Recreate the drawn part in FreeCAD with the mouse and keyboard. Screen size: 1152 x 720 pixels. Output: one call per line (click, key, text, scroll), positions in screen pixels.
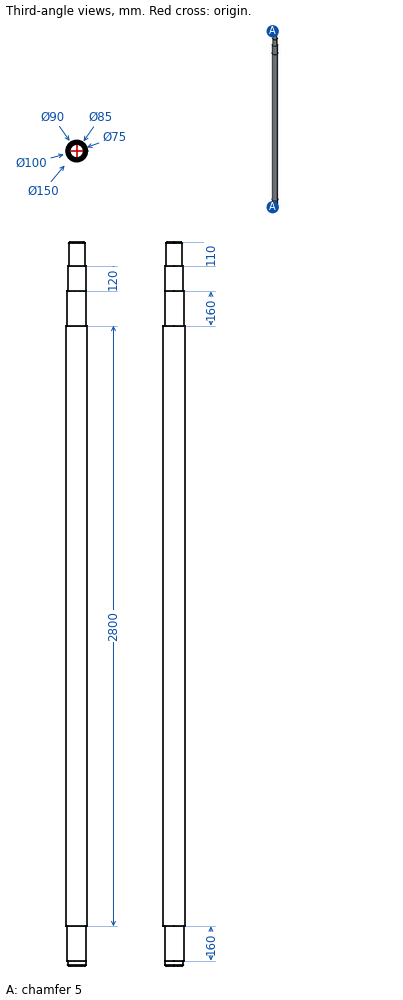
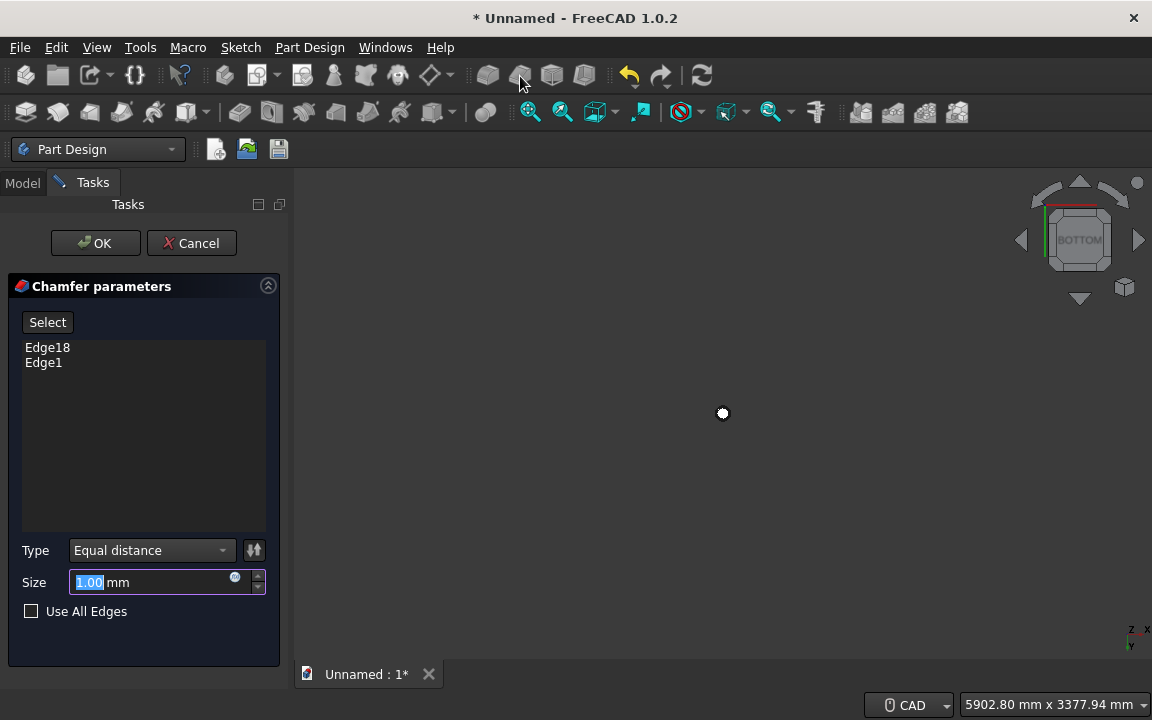
text(5)
key(Tab)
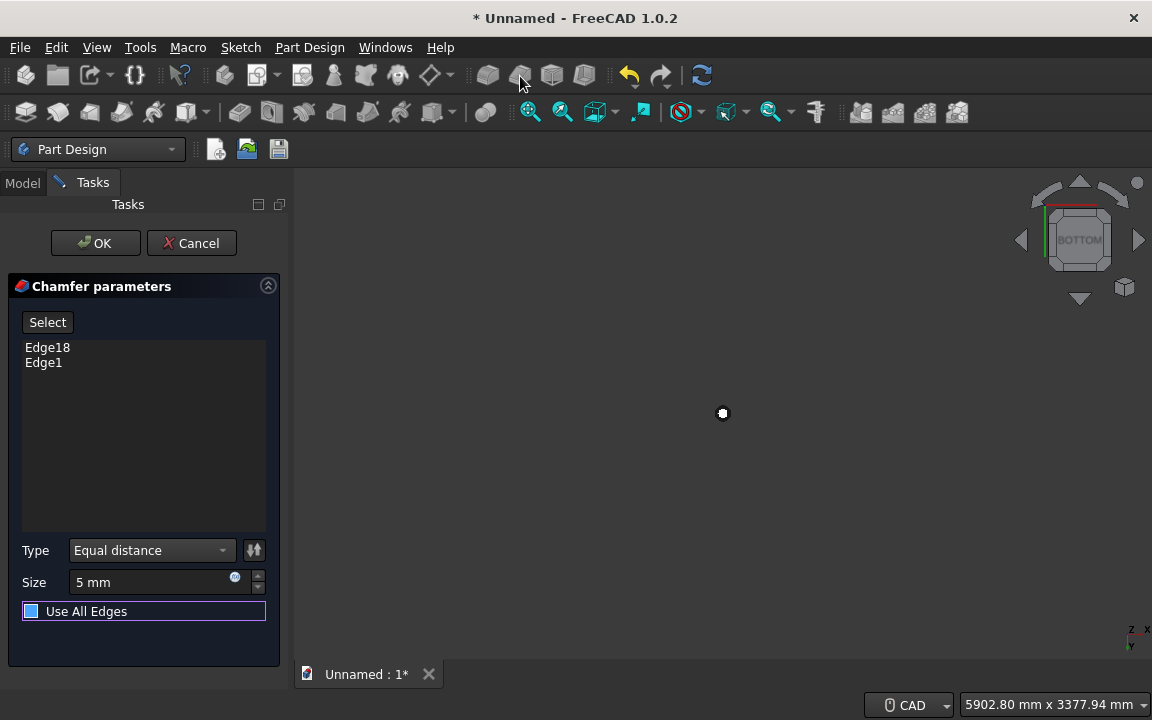
click(96, 243)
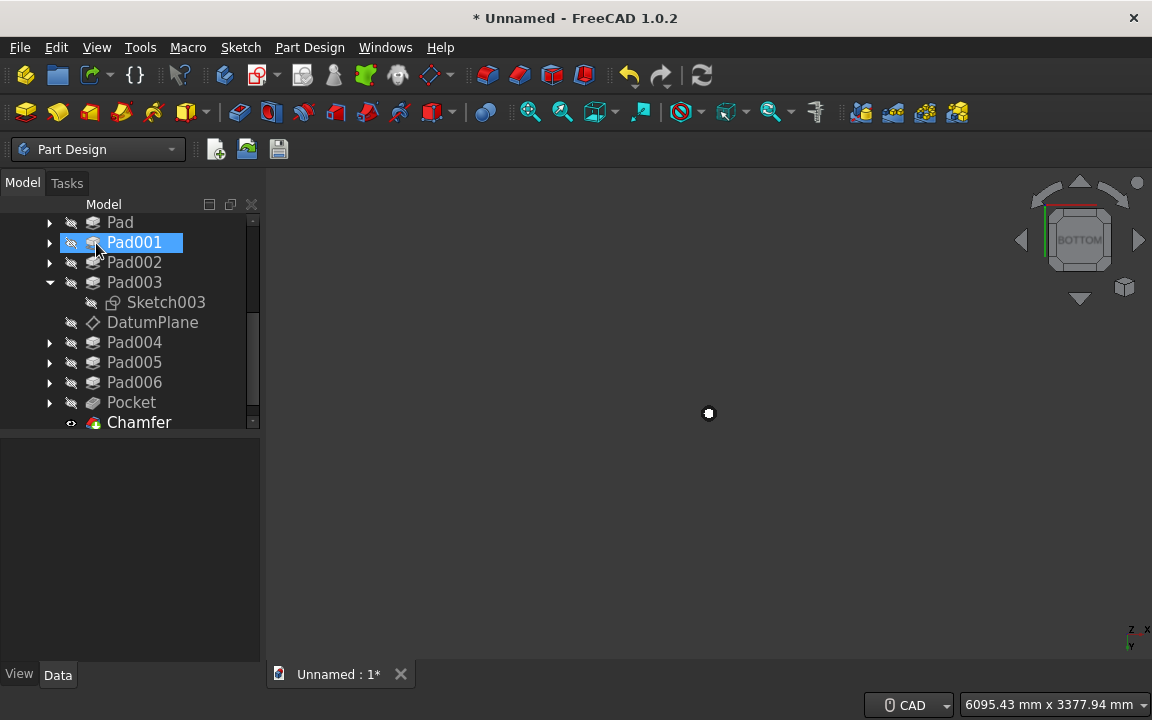
key(0)